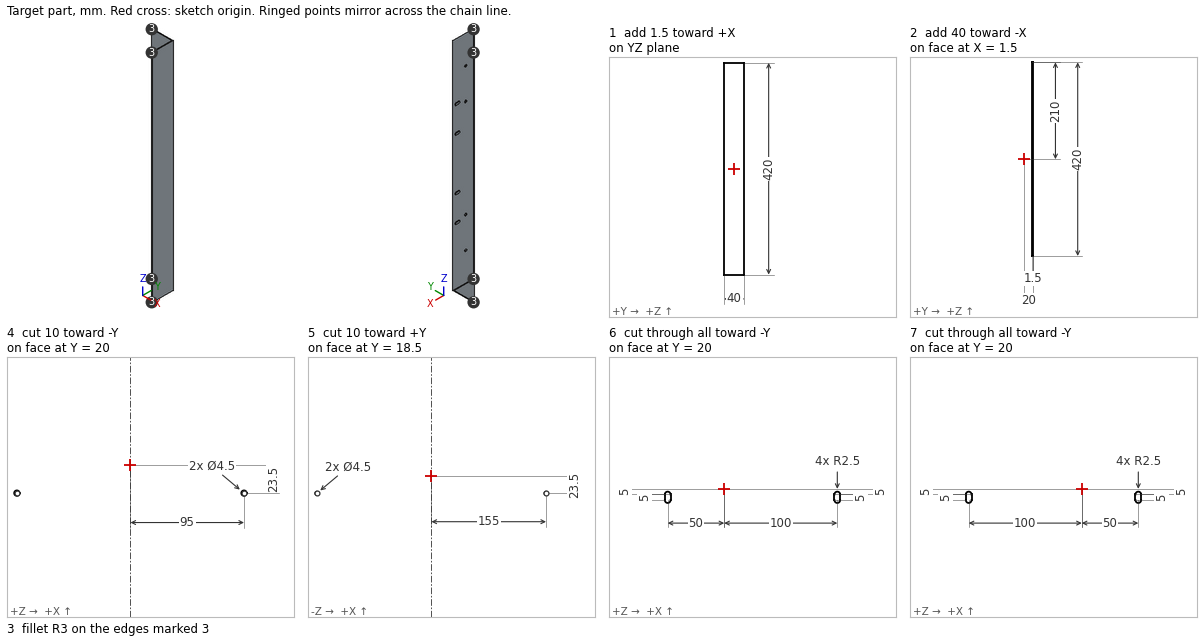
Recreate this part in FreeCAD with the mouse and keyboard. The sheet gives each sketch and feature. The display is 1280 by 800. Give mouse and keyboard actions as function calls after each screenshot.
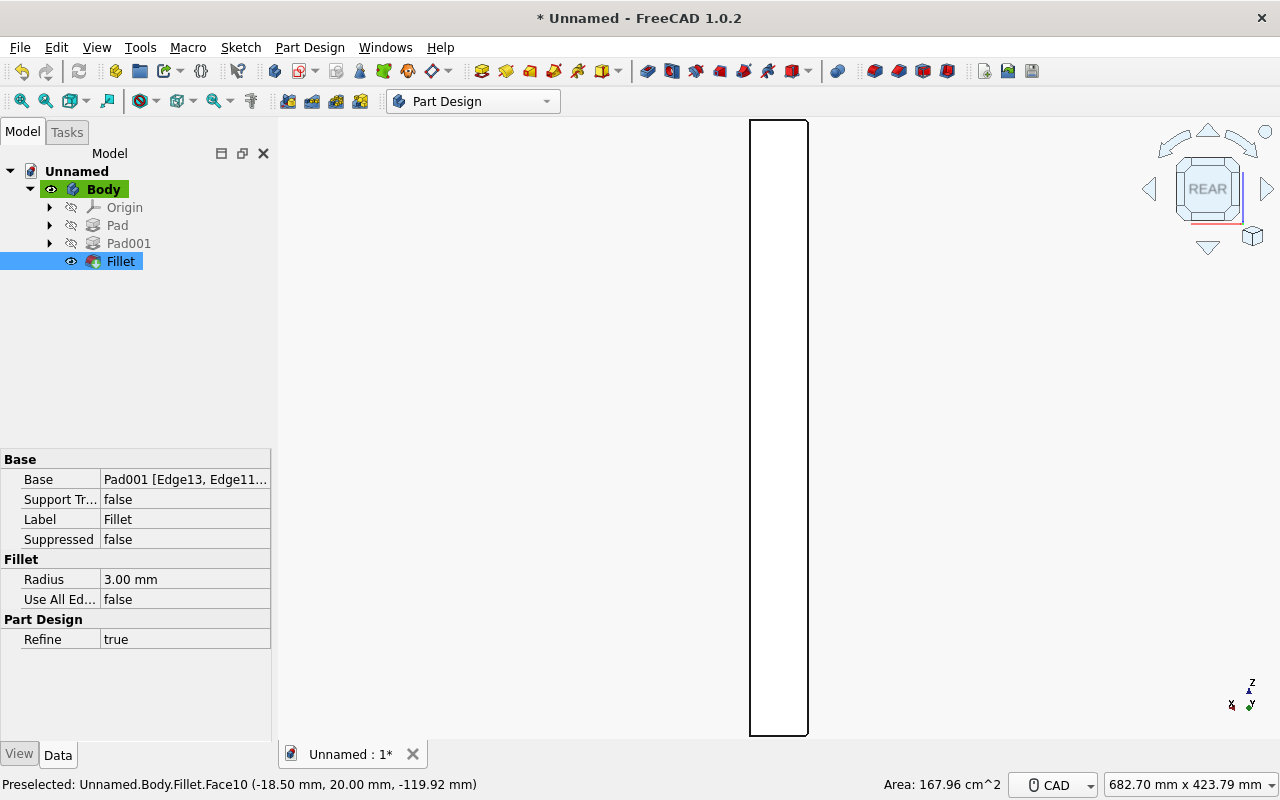
click(300, 72)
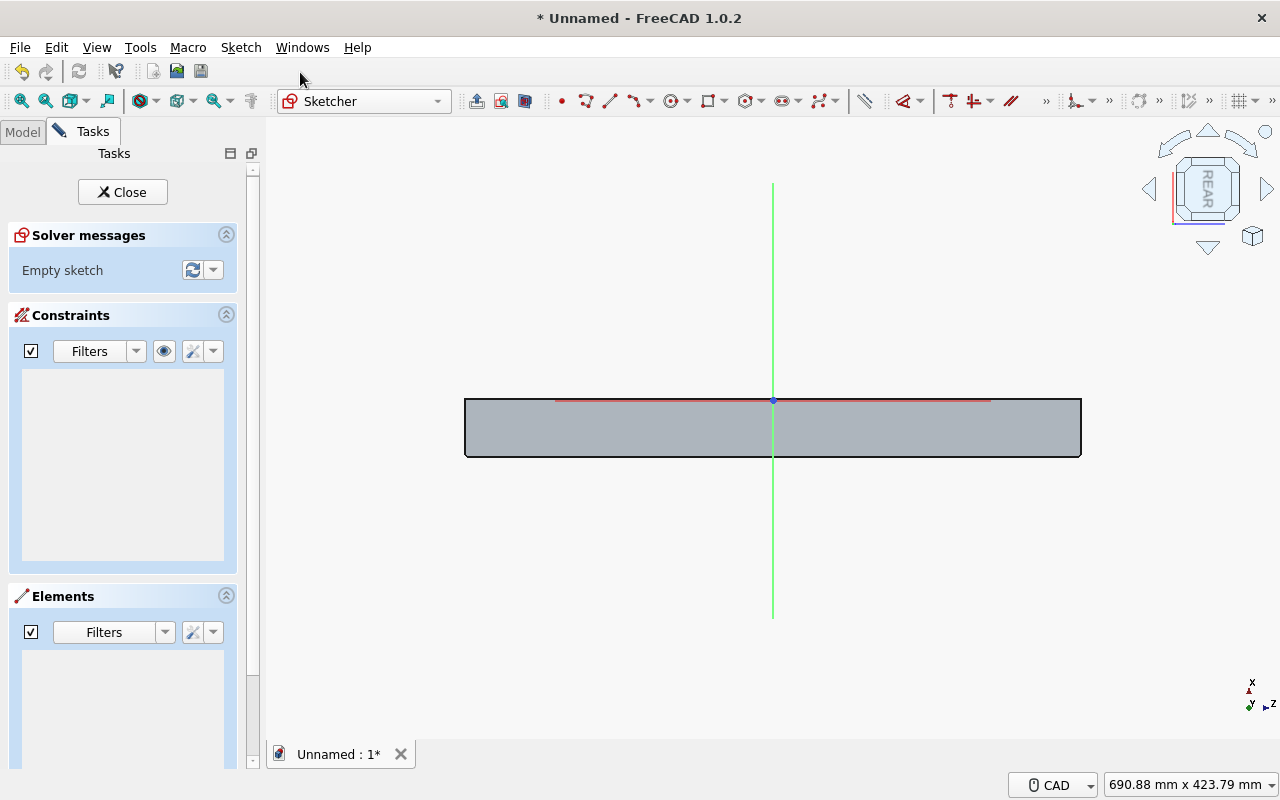
scroll(829, 413, up, 4)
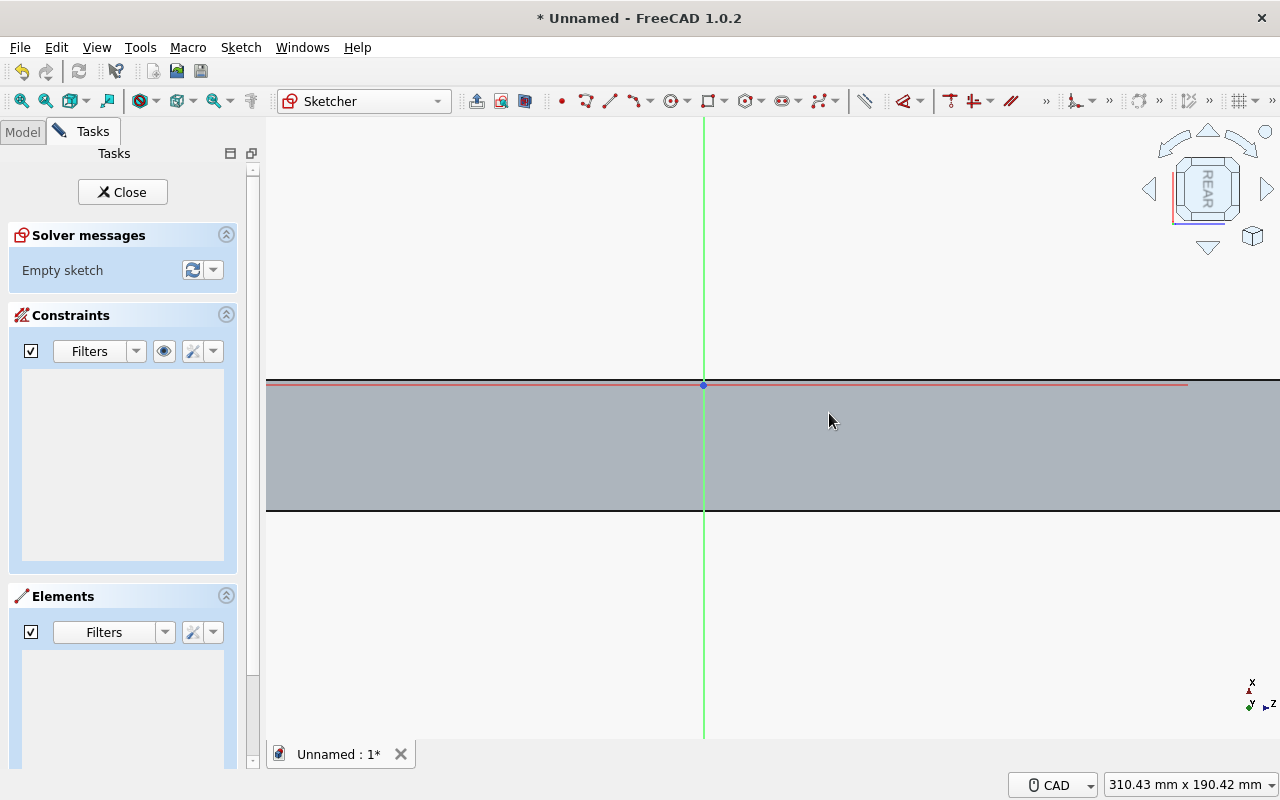
click(672, 102)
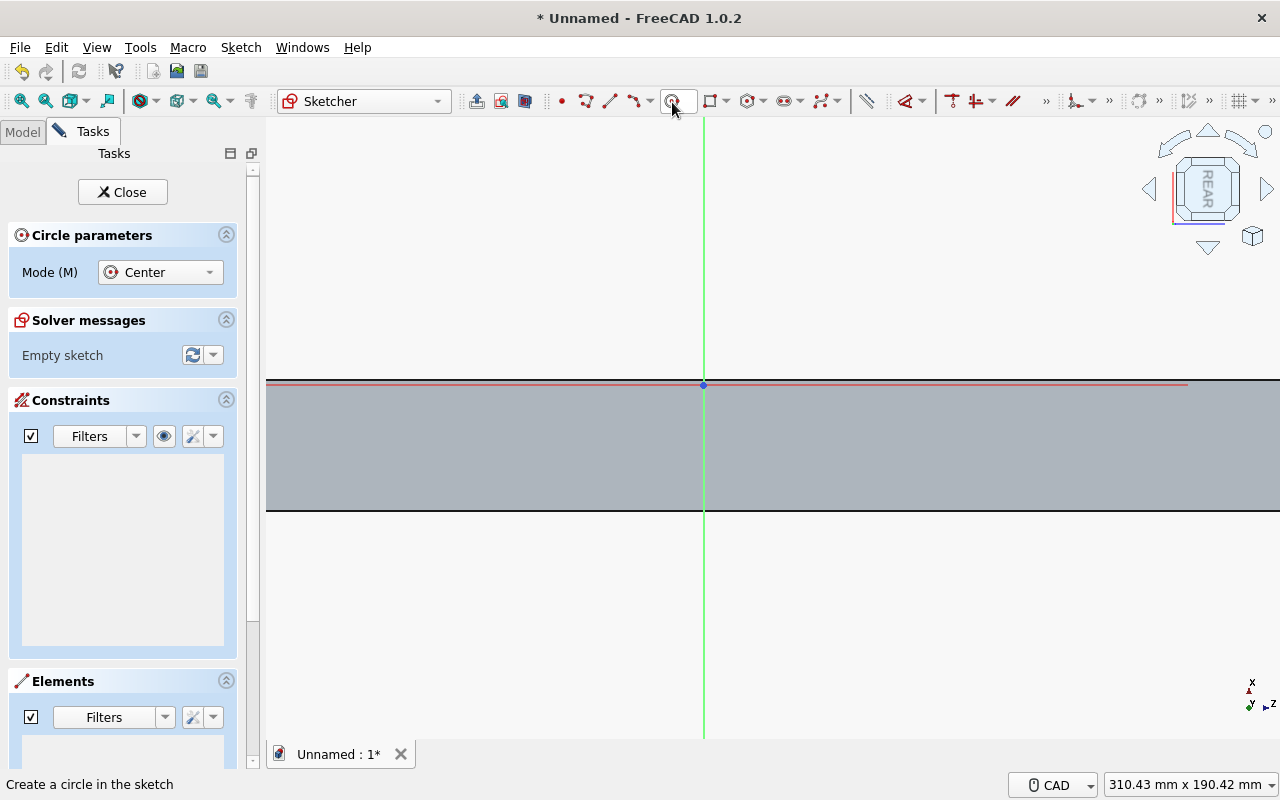
scroll(1014, 462, up, 6)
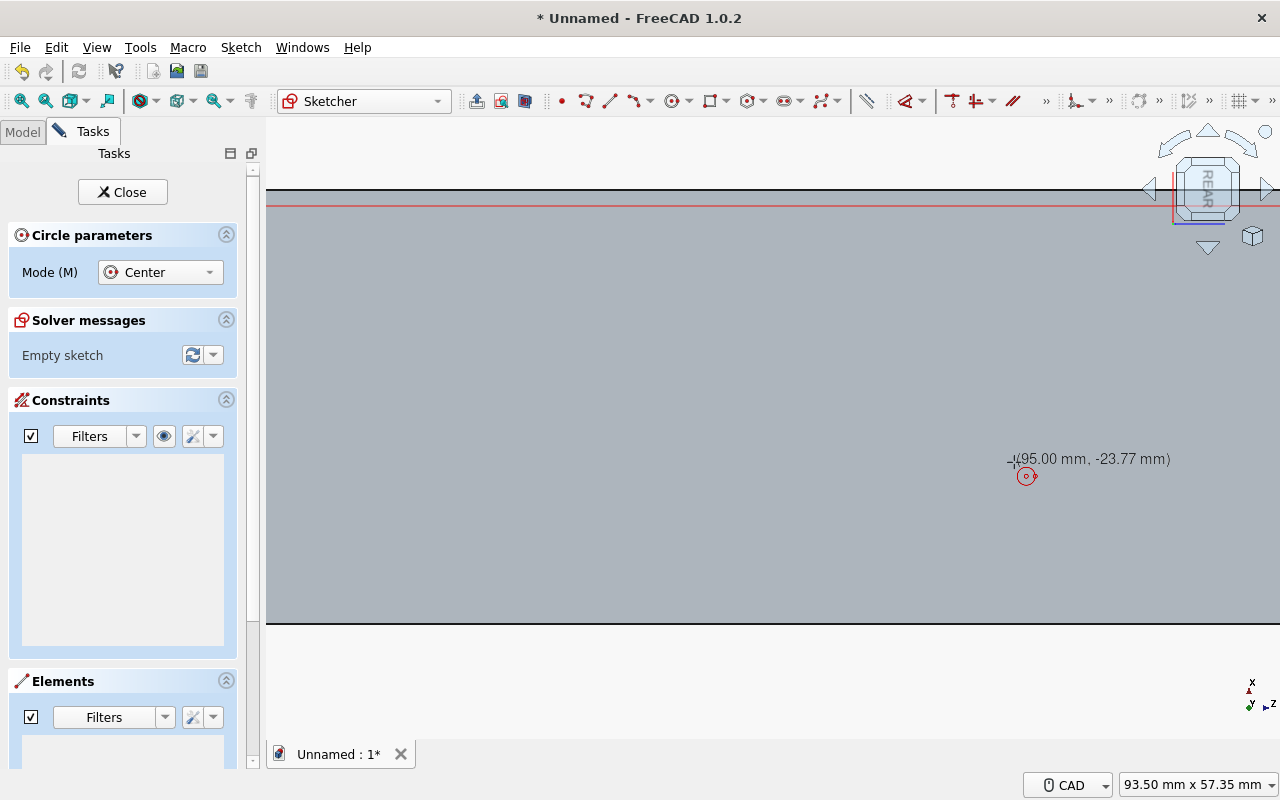
click(1012, 461)
click(1030, 444)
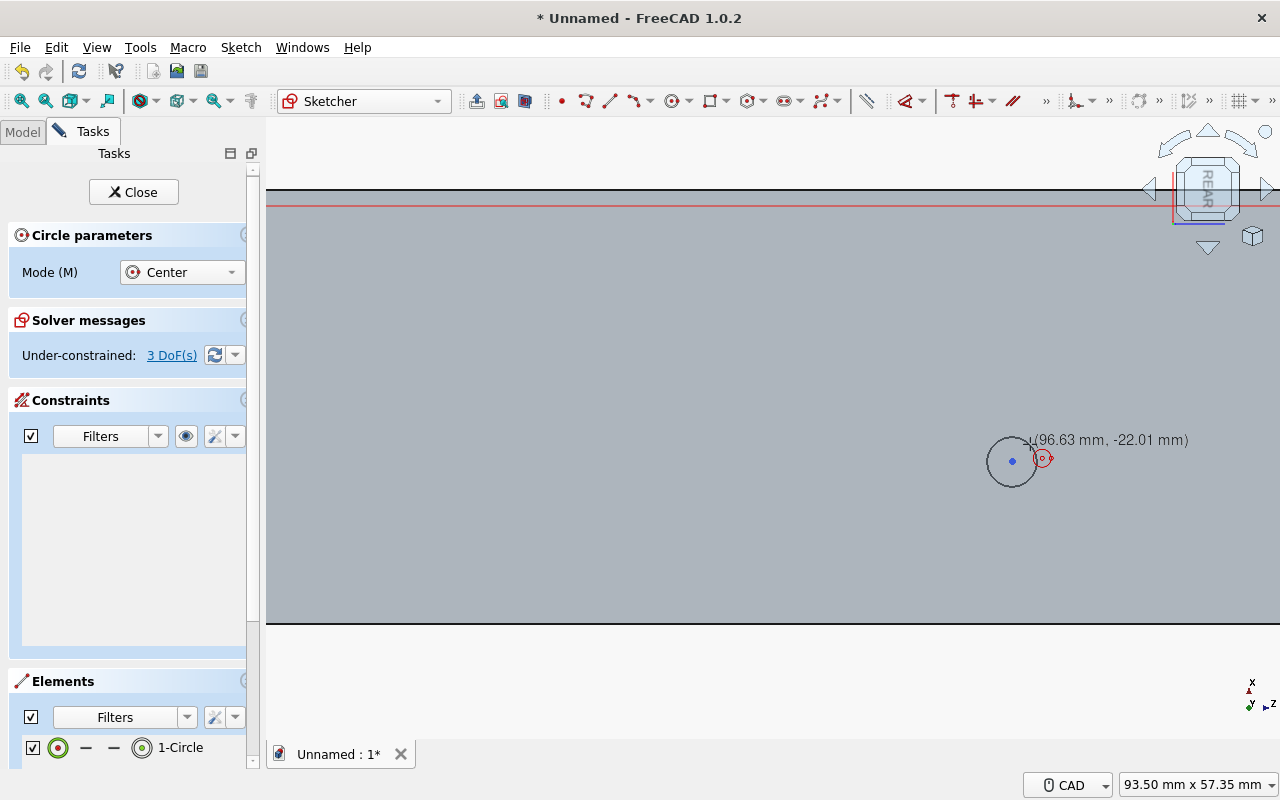
scroll(1016, 463, down, 6)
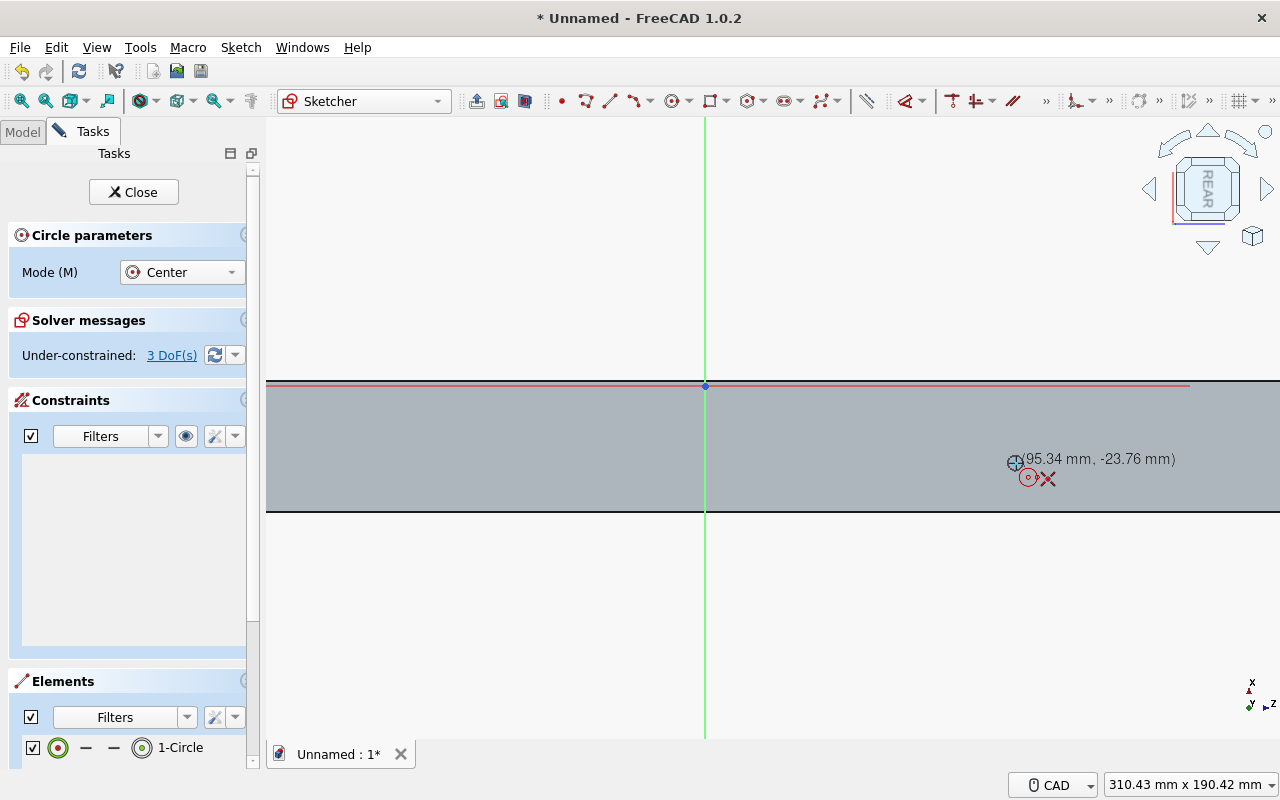
scroll(395, 463, up, 6)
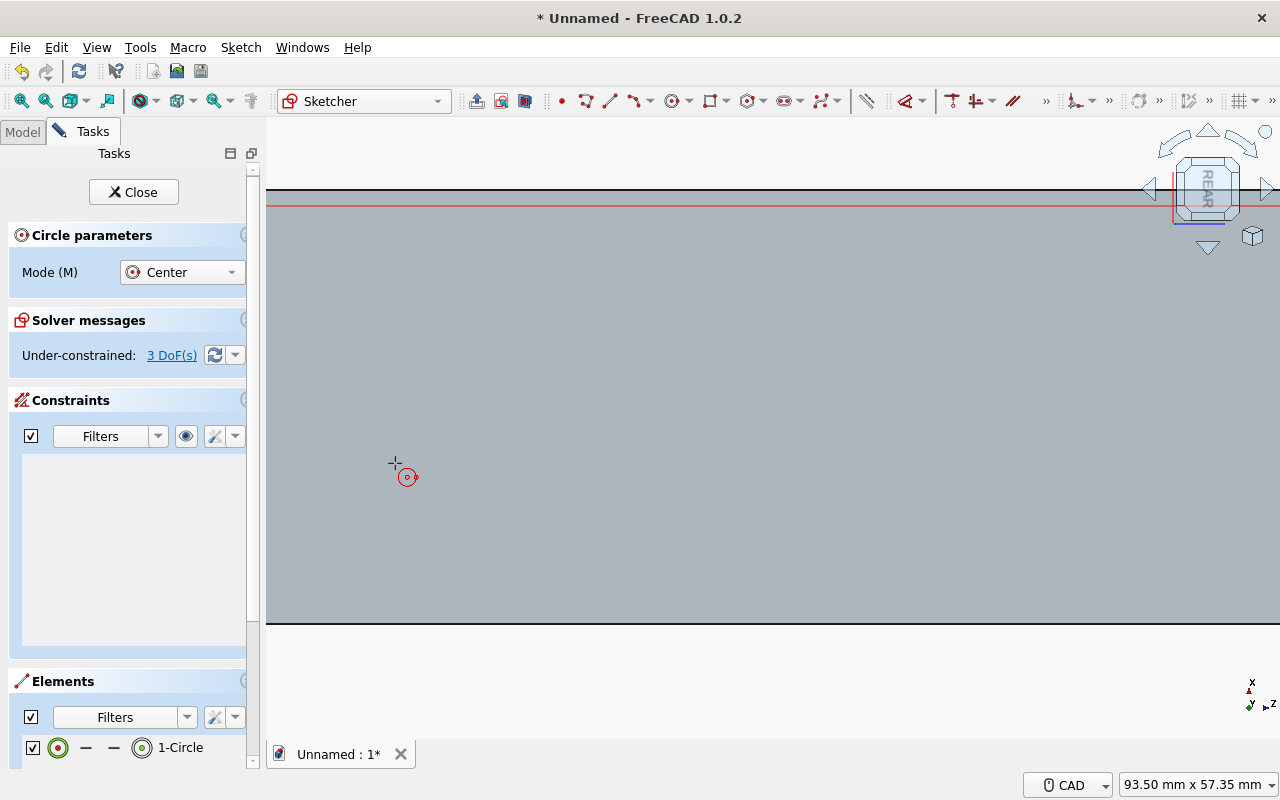
click(394, 461)
click(411, 444)
key(Escape)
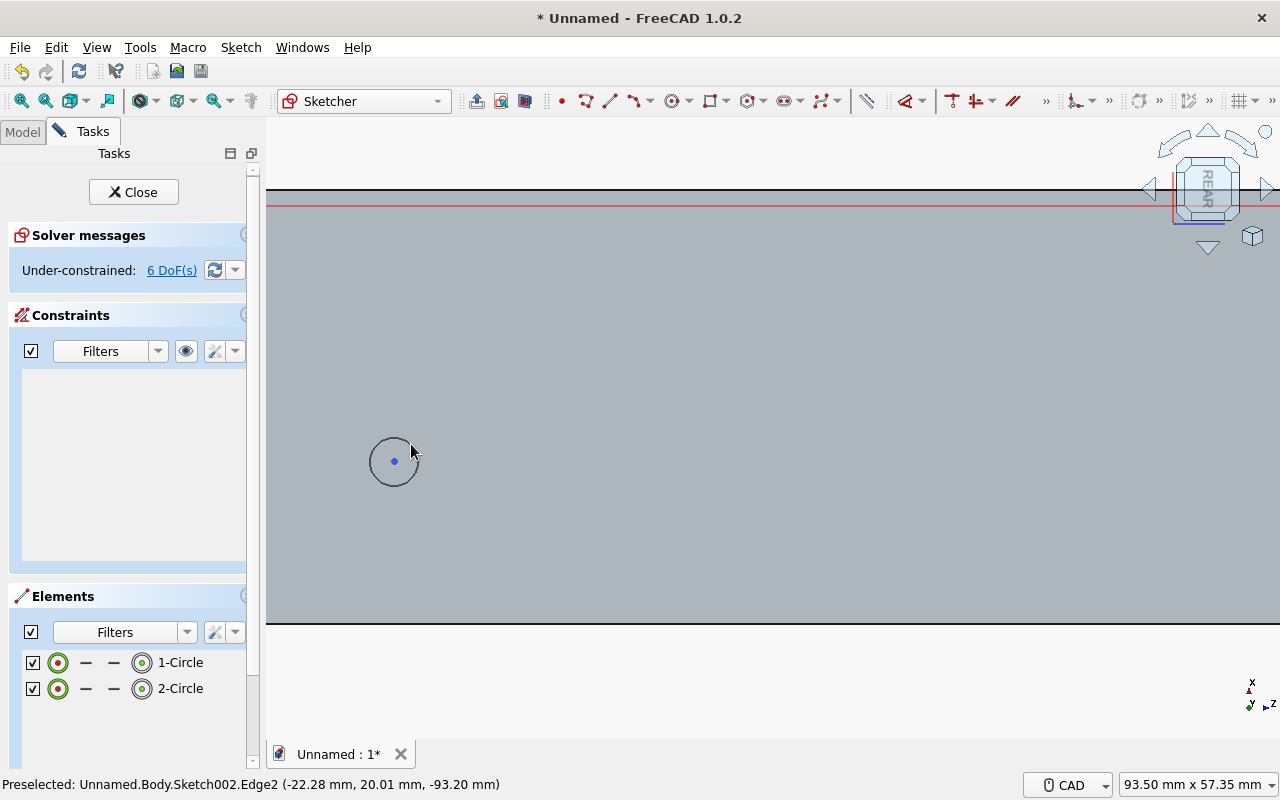
scroll(394, 463, down, 6)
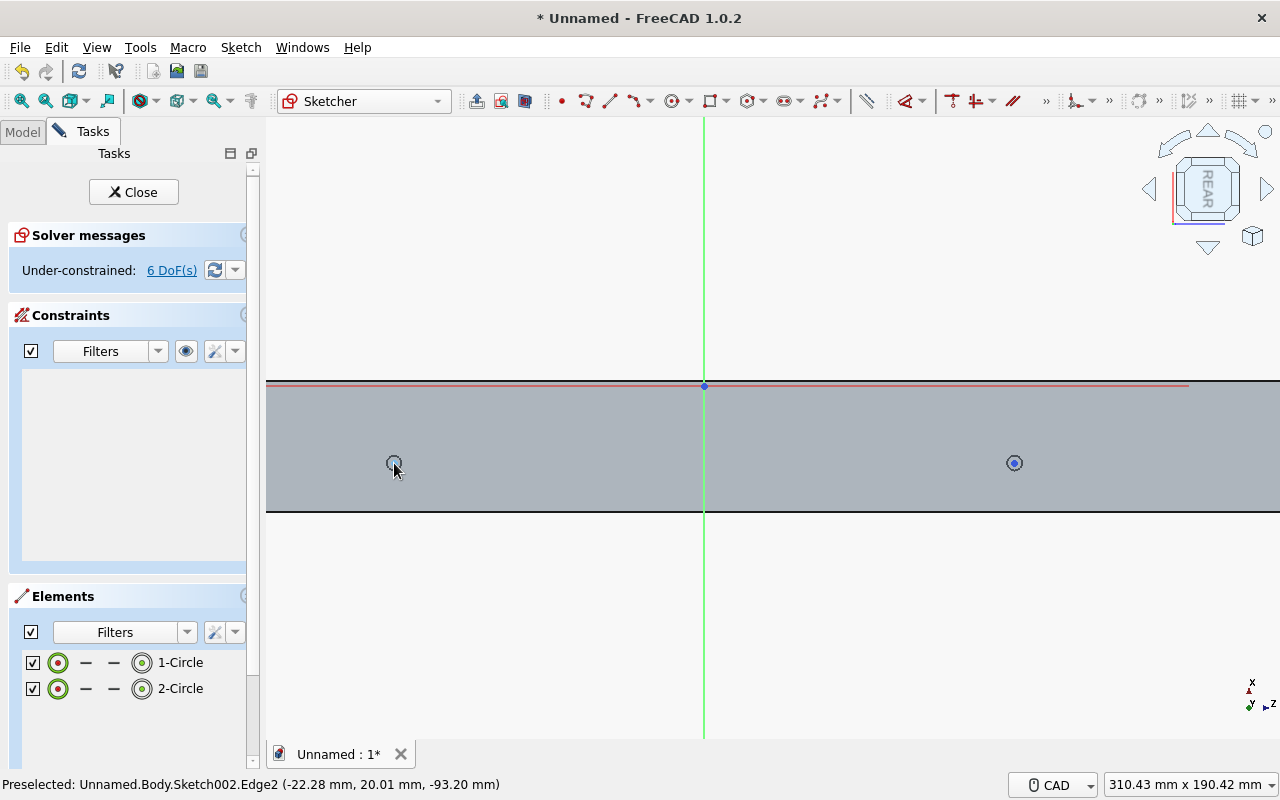
scroll(1020, 458, up, 4)